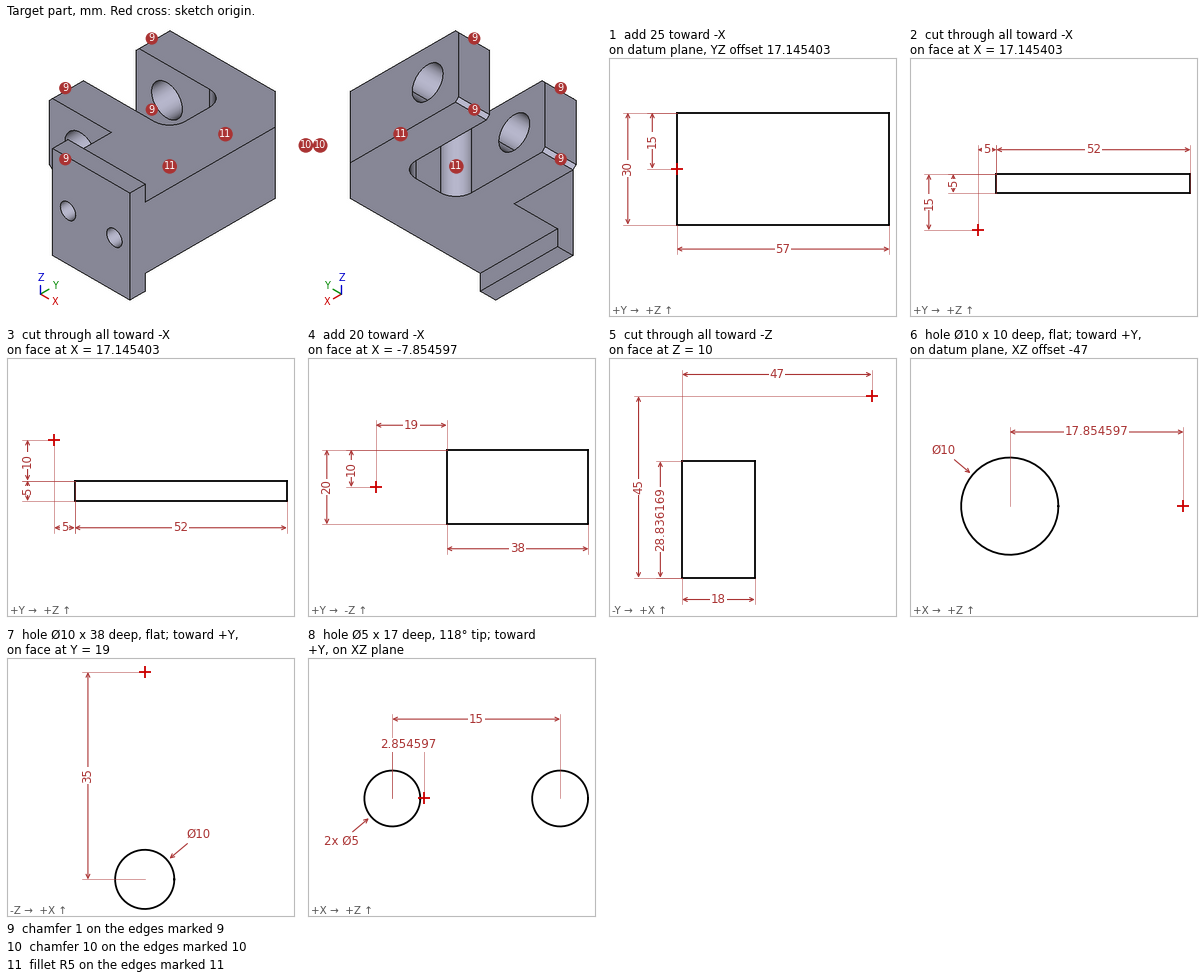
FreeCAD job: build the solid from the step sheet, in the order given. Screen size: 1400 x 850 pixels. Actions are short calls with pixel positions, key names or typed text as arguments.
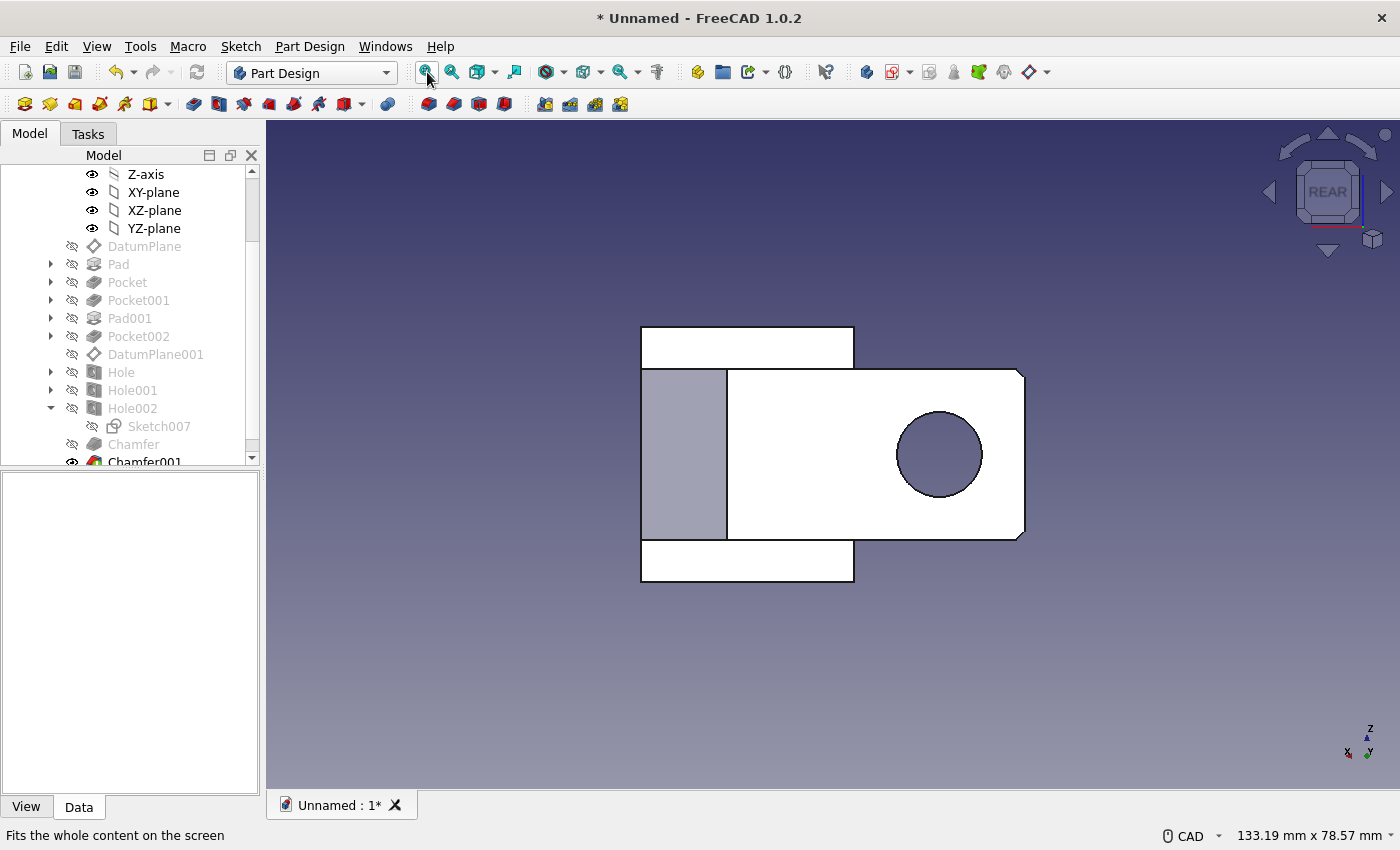
key(6)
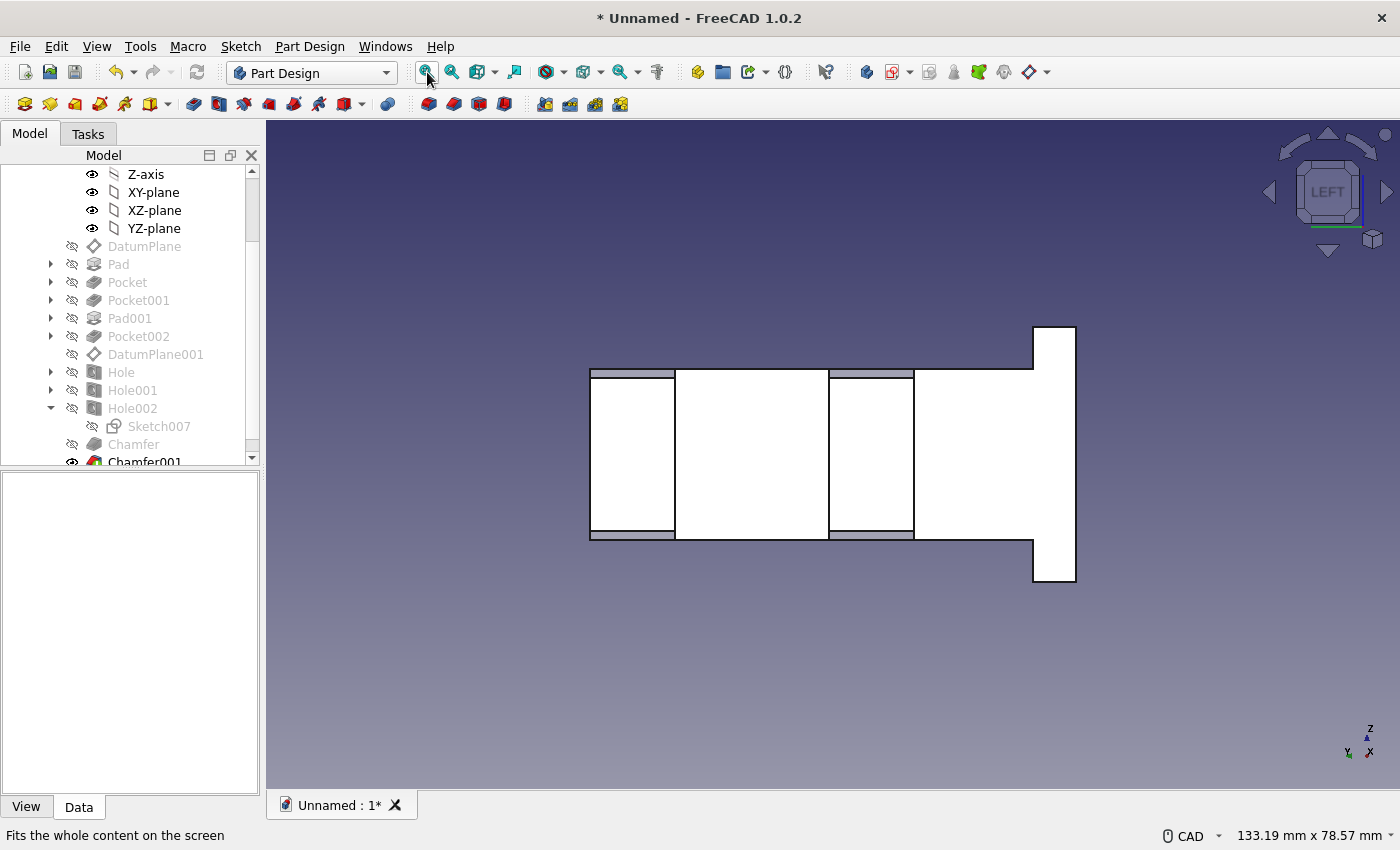
key(v)
key(f)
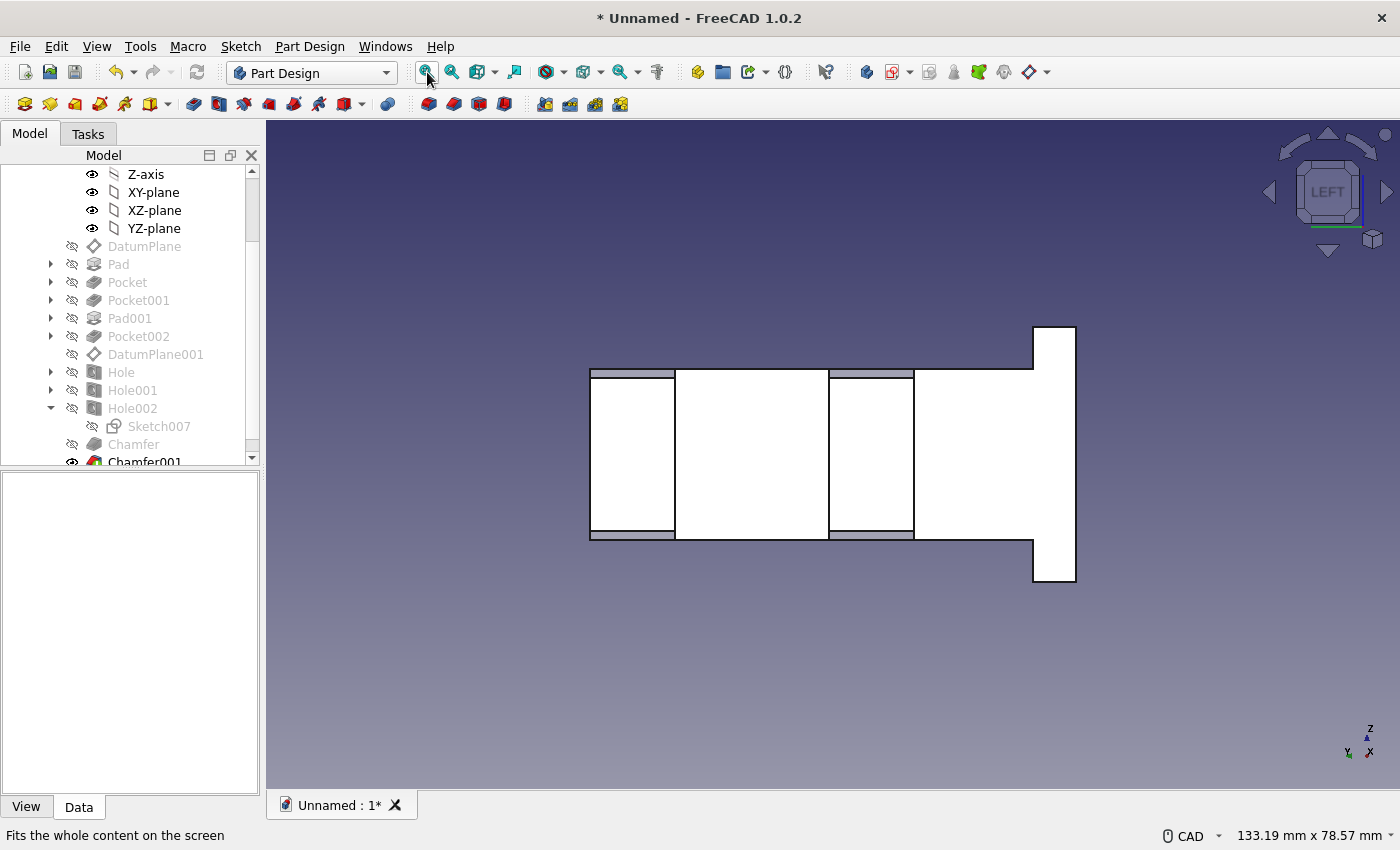
key(v)
key(3)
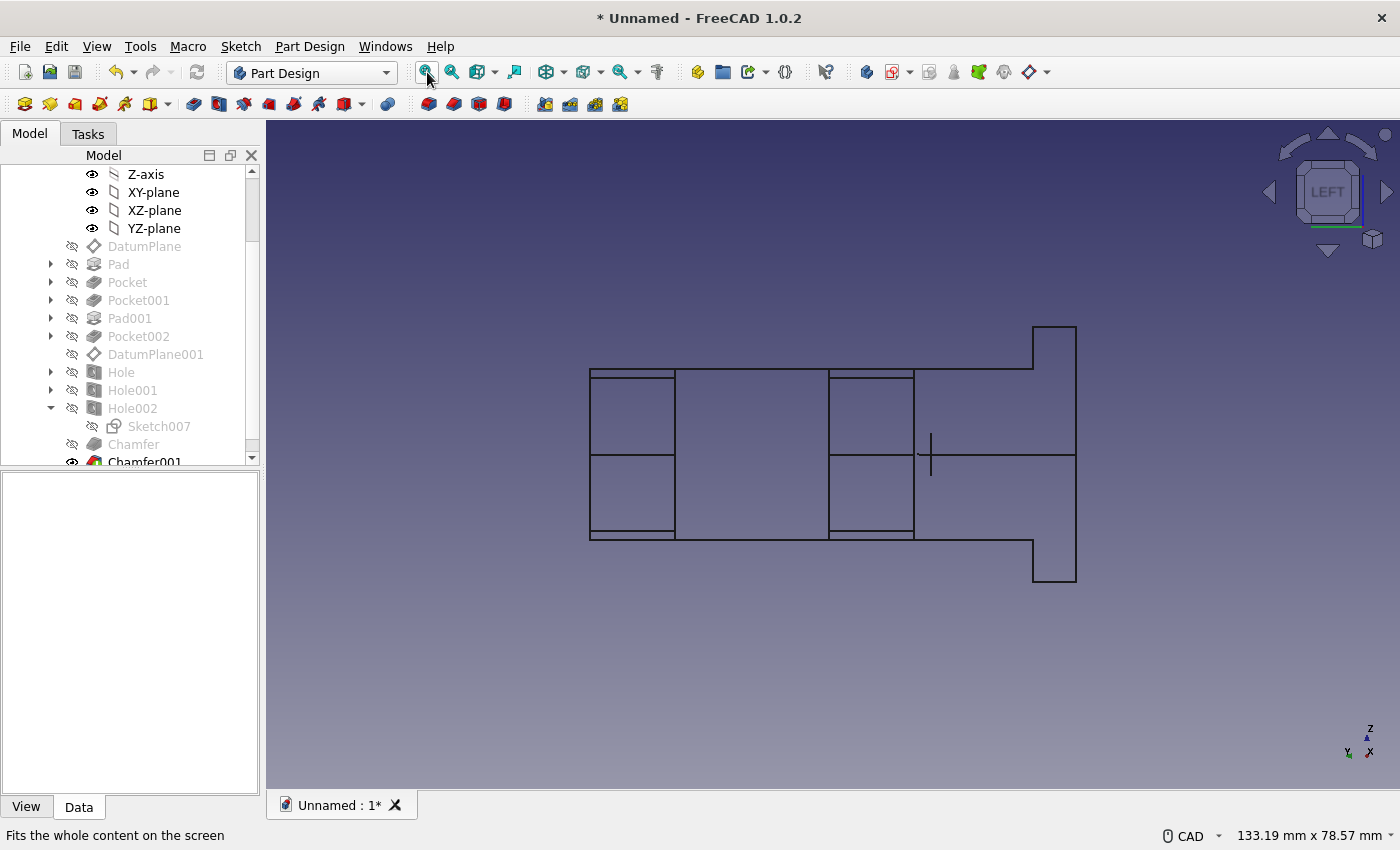
key(0)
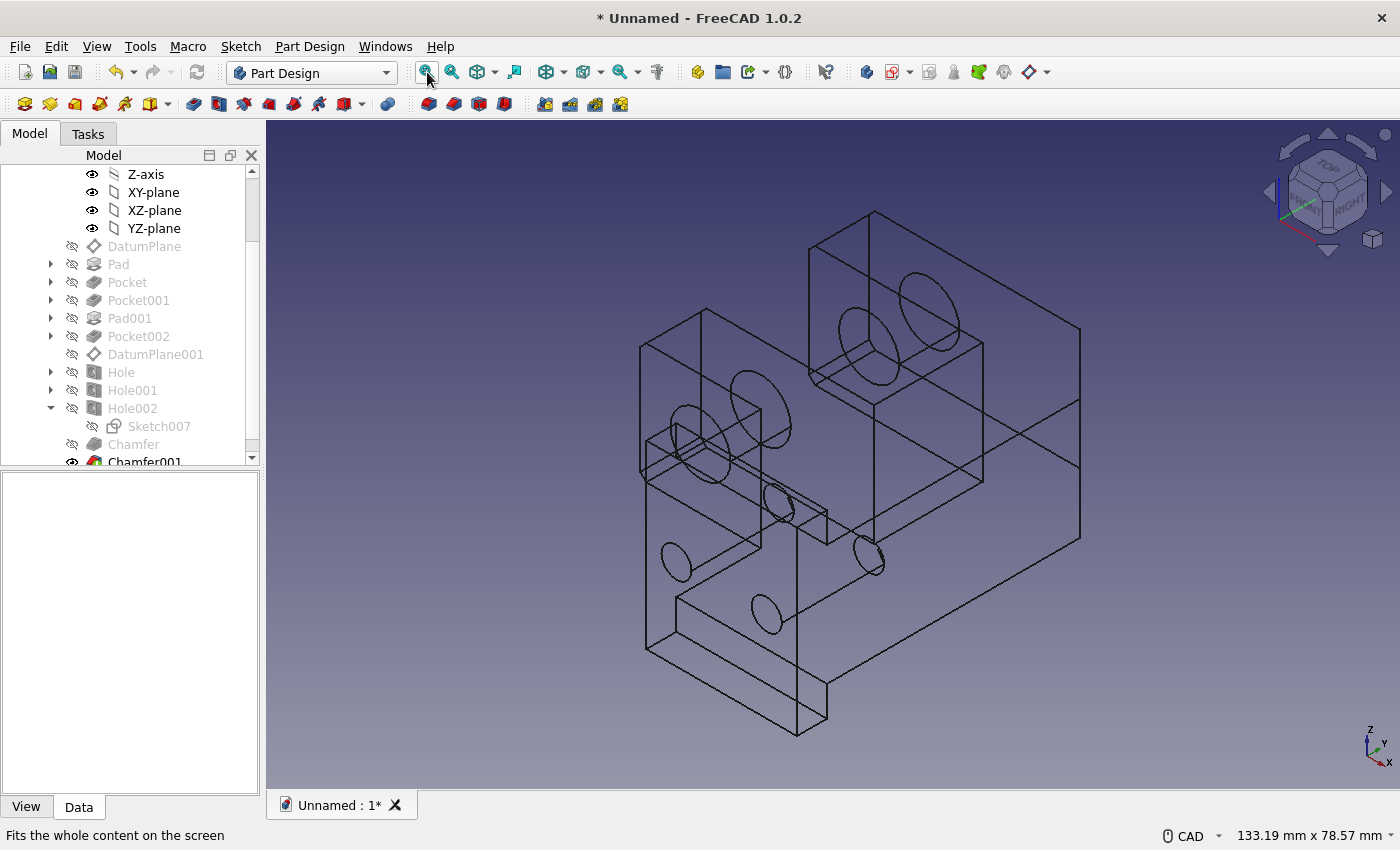
click(983, 411)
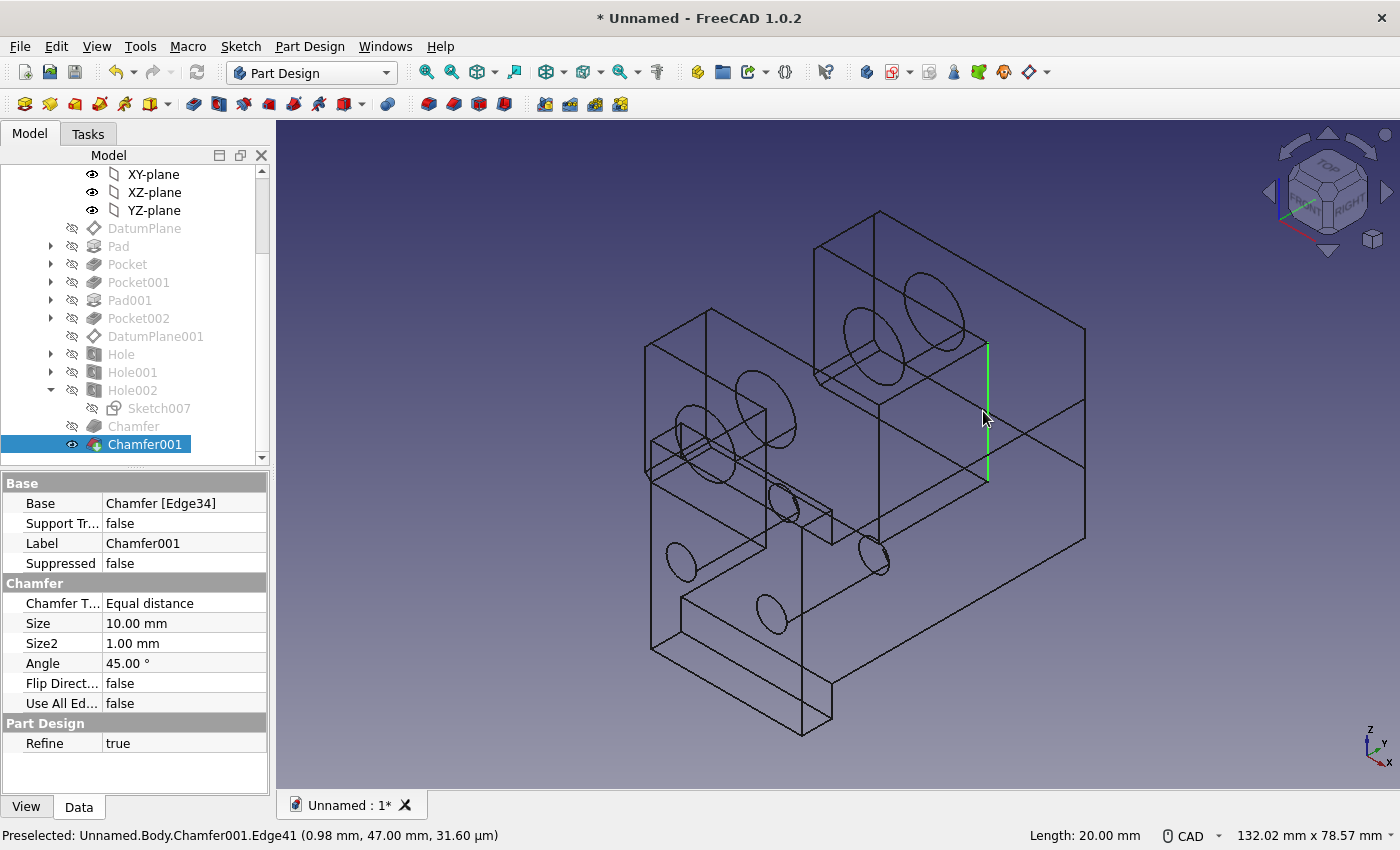
click(879, 474, ctrl)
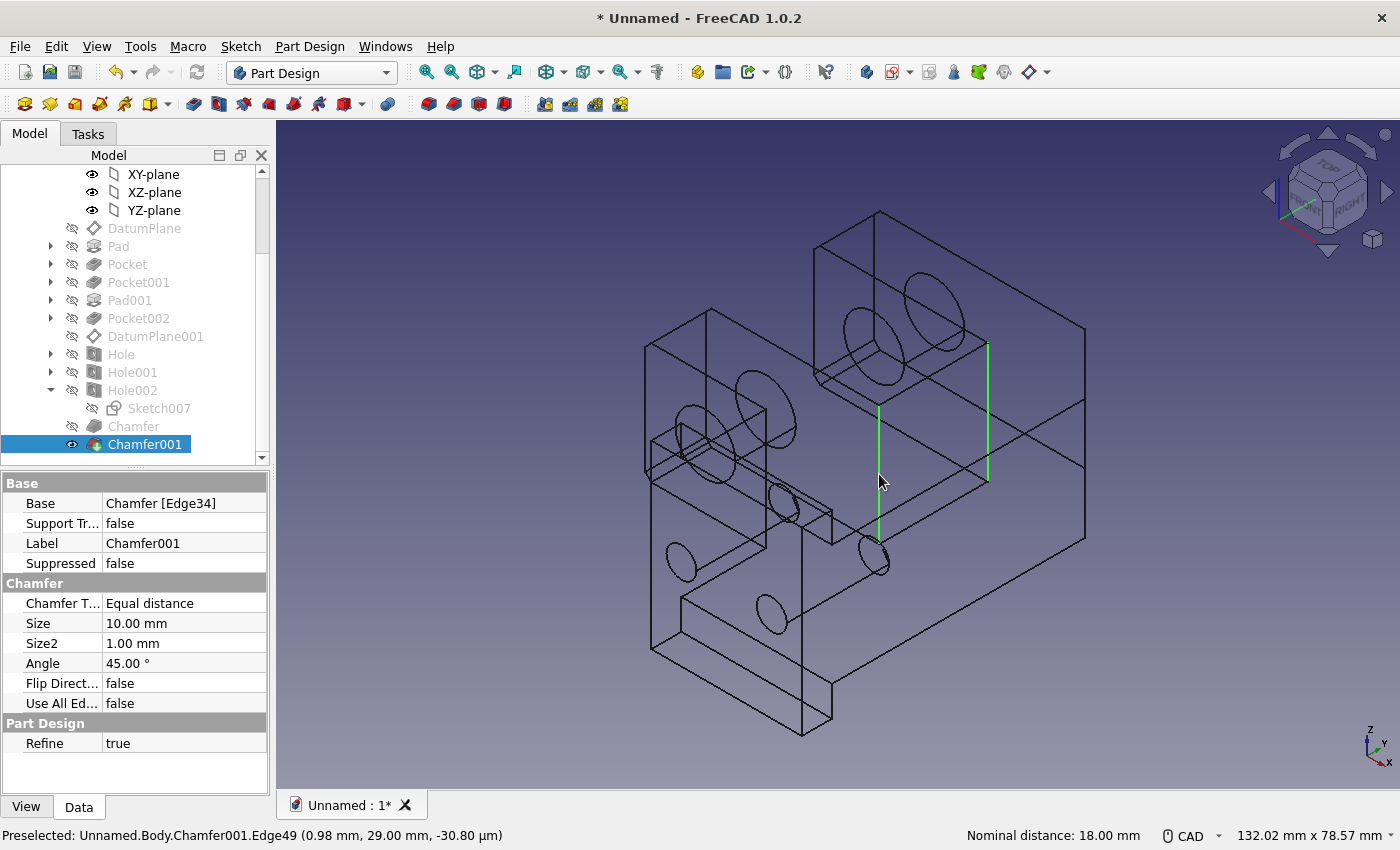
key(v)
key(1)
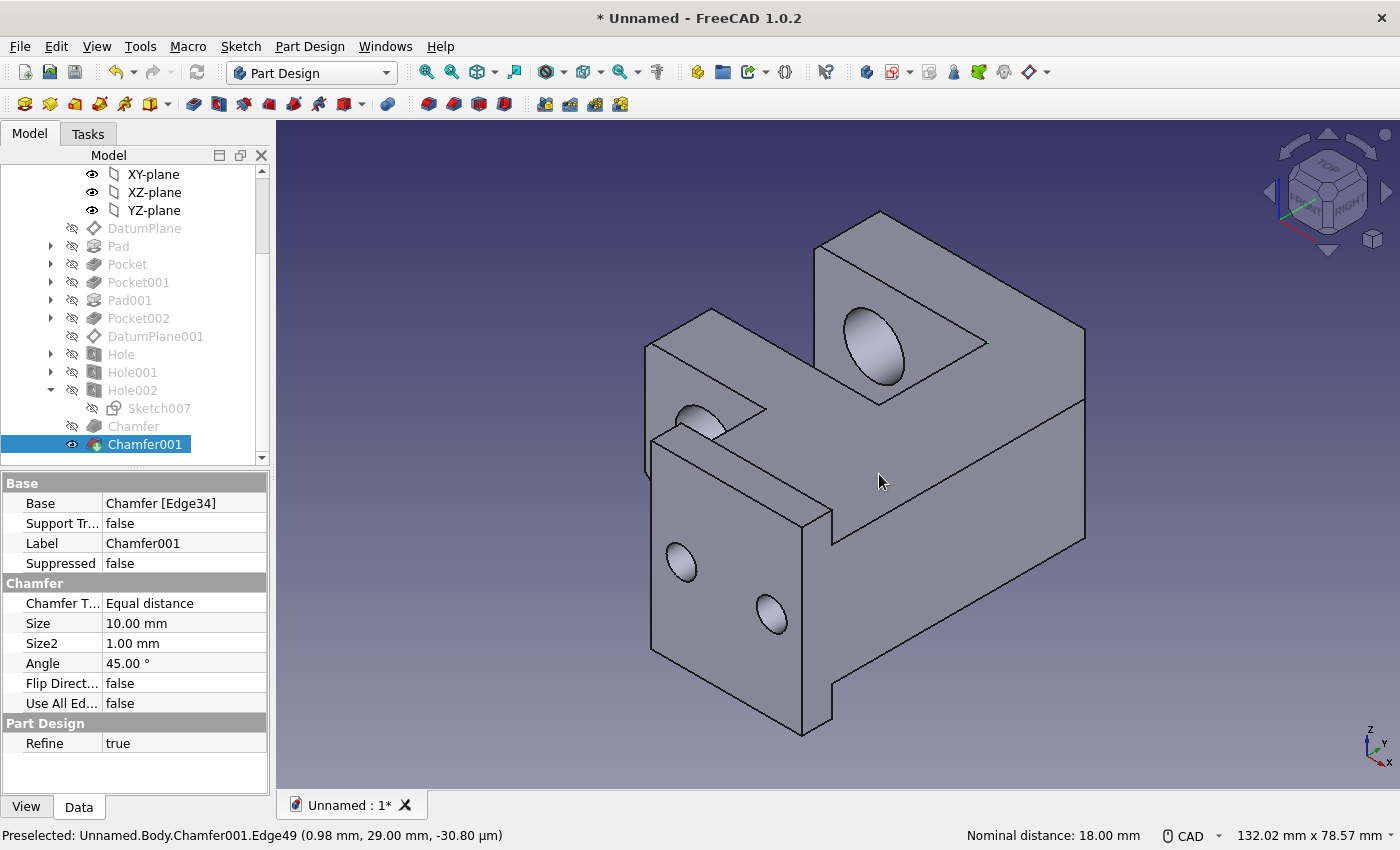
click(429, 104)